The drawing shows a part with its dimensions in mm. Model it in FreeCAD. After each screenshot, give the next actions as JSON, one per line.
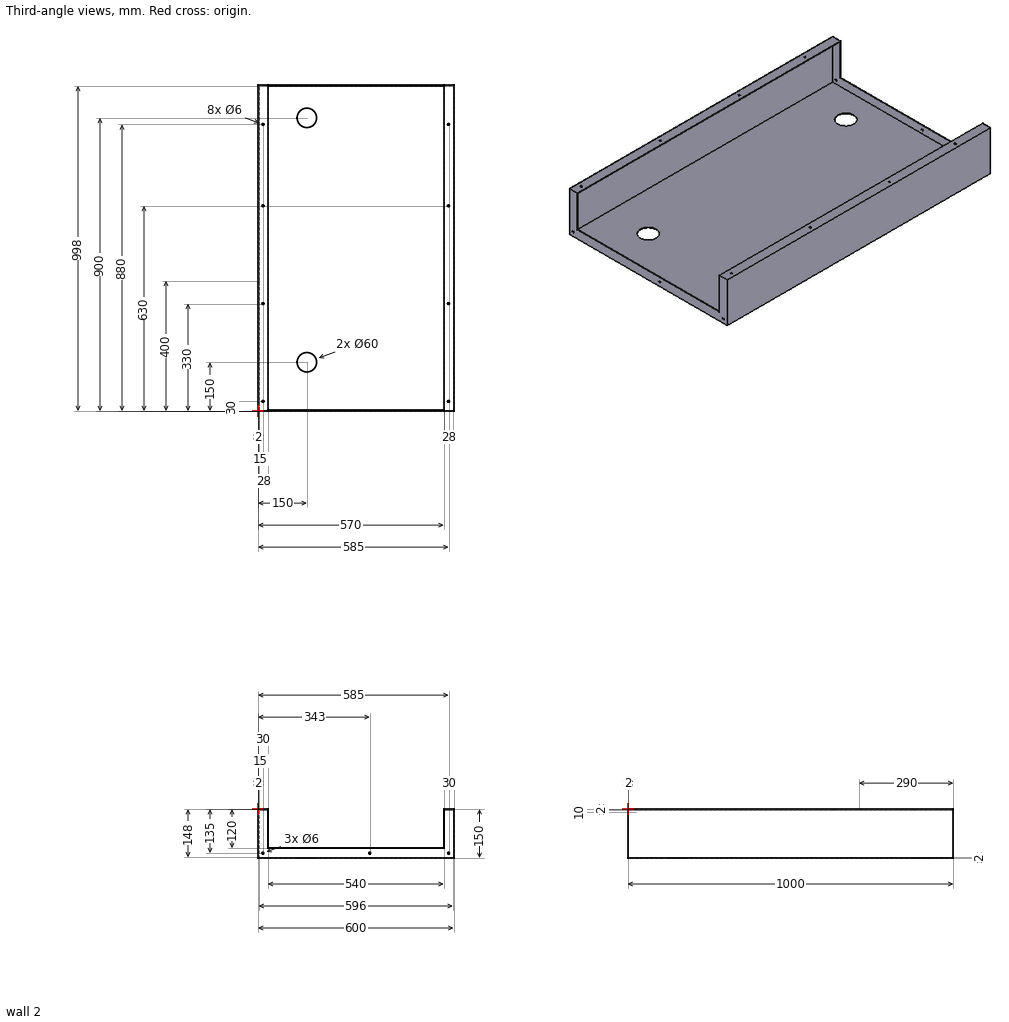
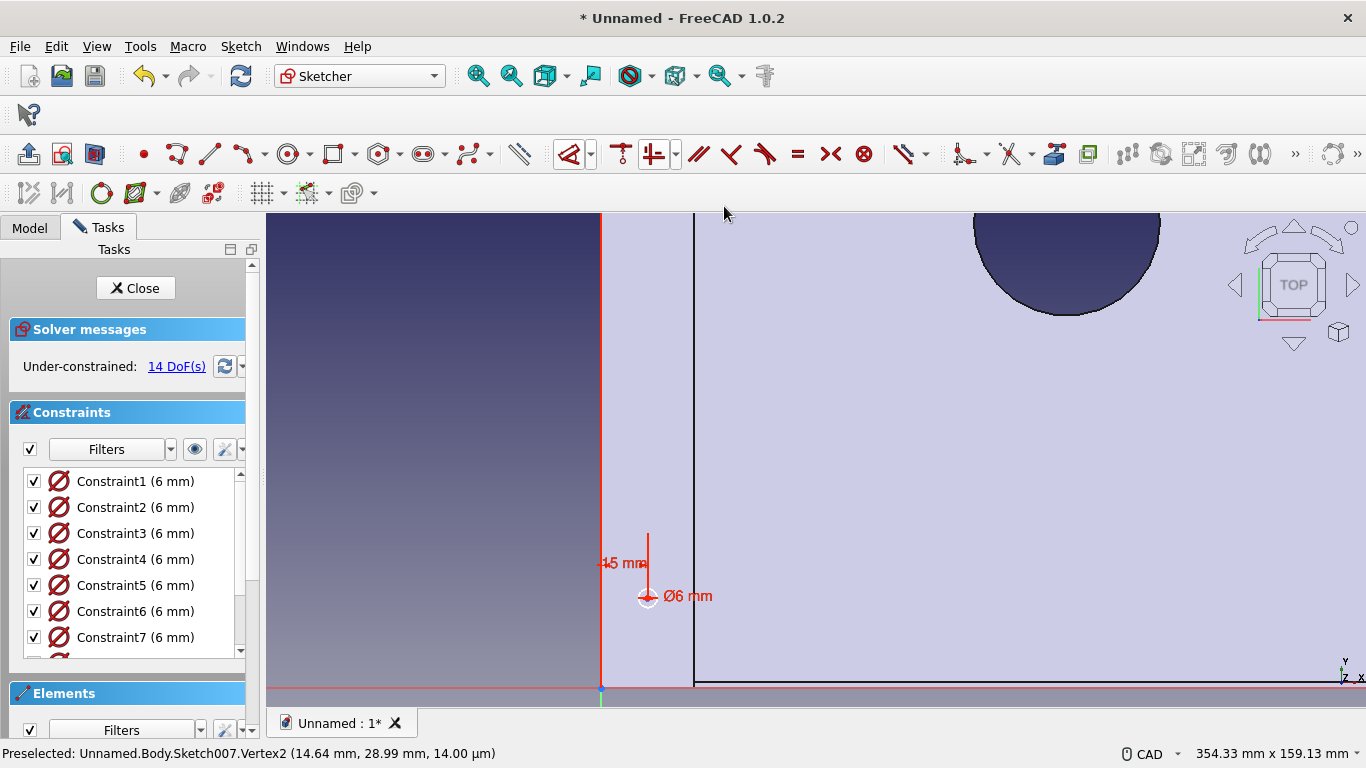
{"action": "left_click", "coordinate": [648, 598]}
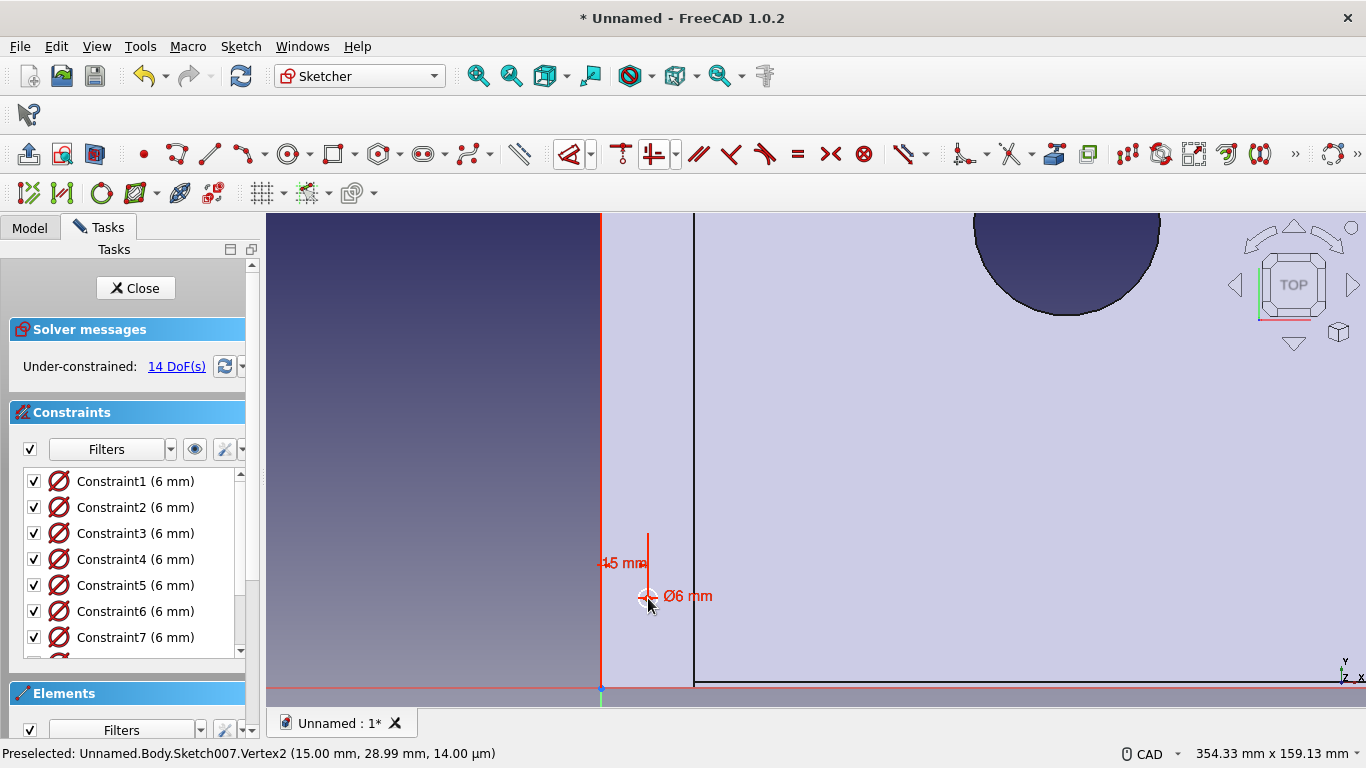
{"action": "left_click", "coordinate": [590, 154]}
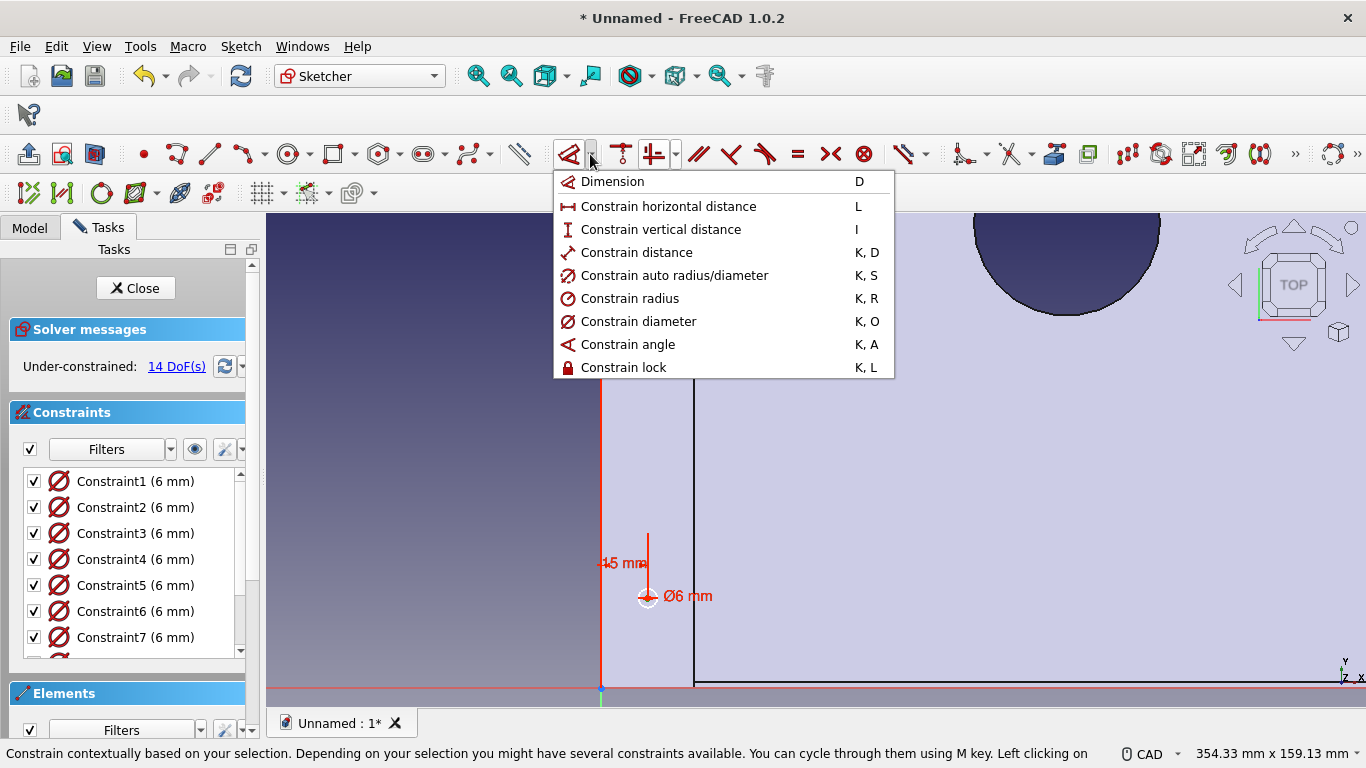
{"action": "left_click", "coordinate": [724, 230]}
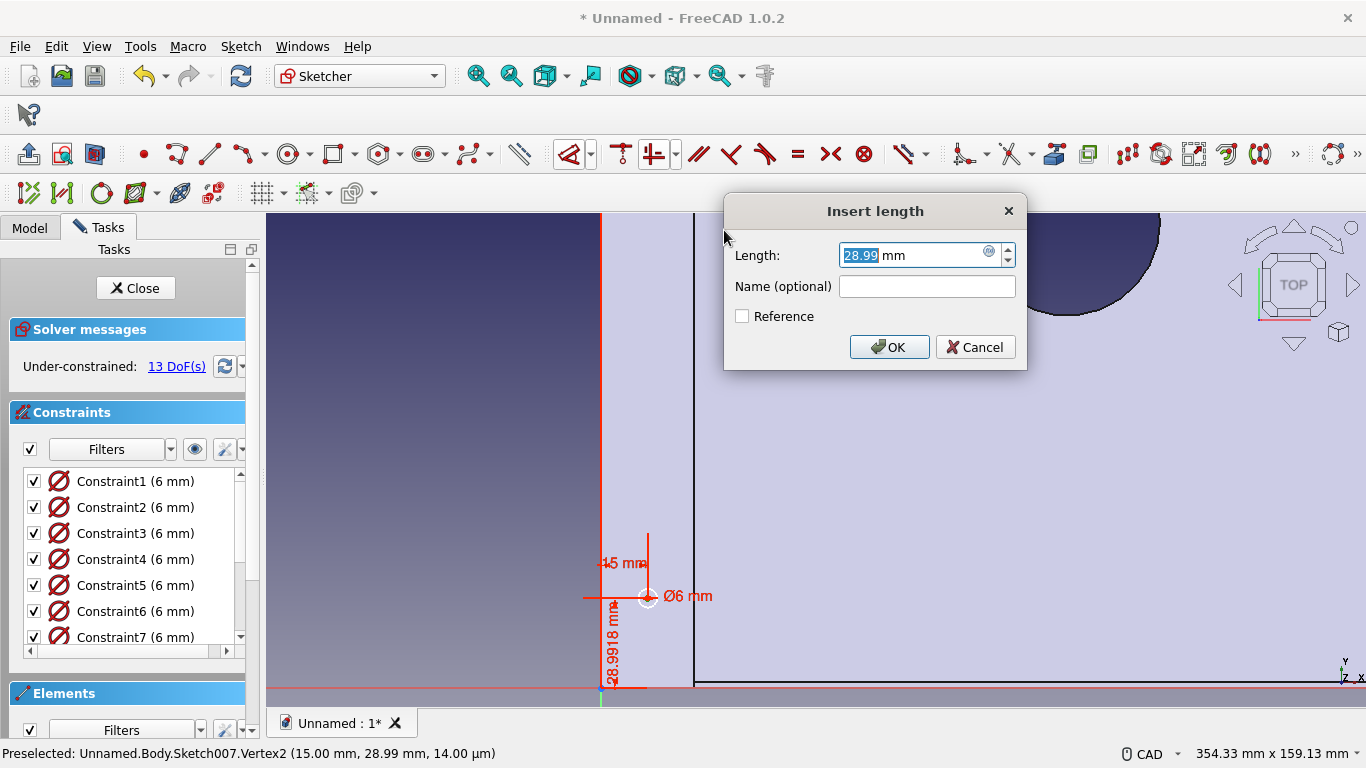
{"action": "type", "text": "30"}
{"action": "key", "text": "Return"}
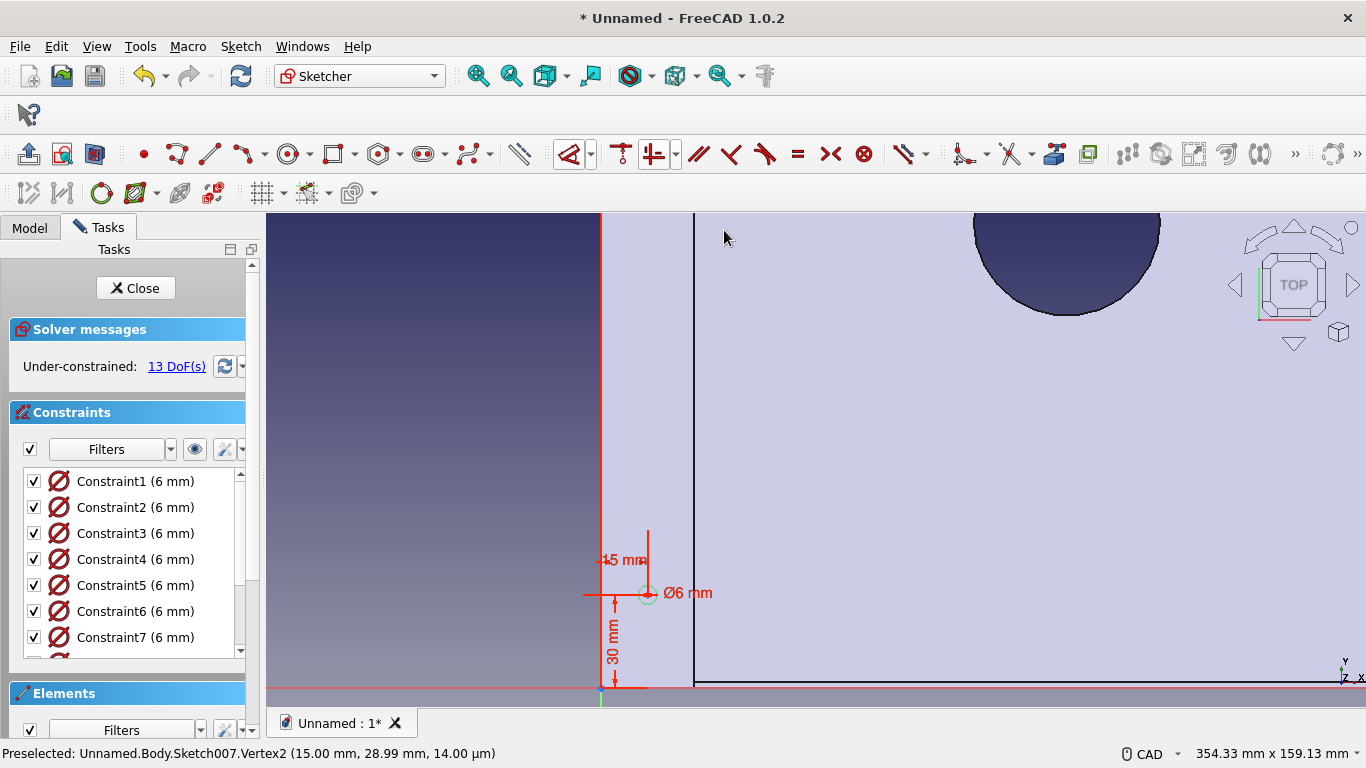
{"action": "scroll", "coordinate": [652, 602], "scroll_direction": "down", "scroll_amount": 11}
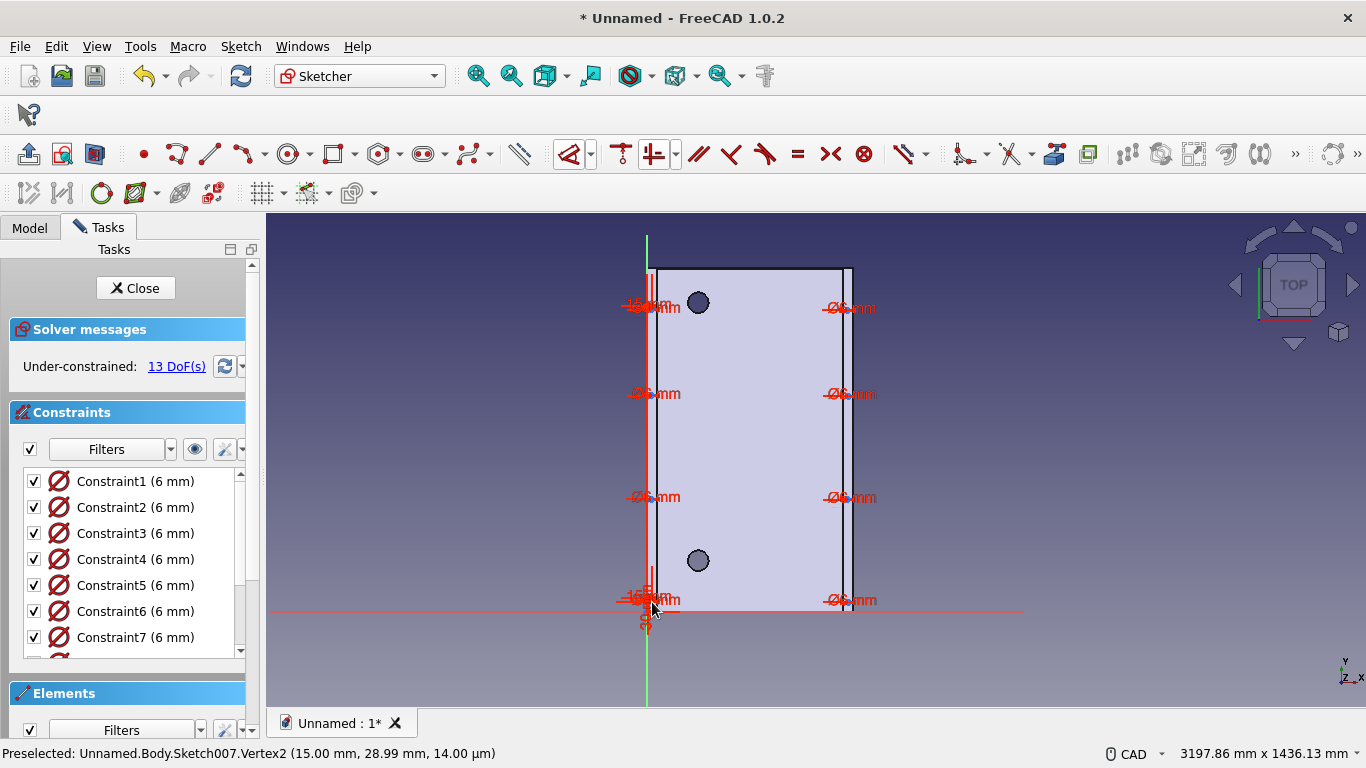
{"action": "scroll", "coordinate": [652, 499], "scroll_direction": "up", "scroll_amount": 11}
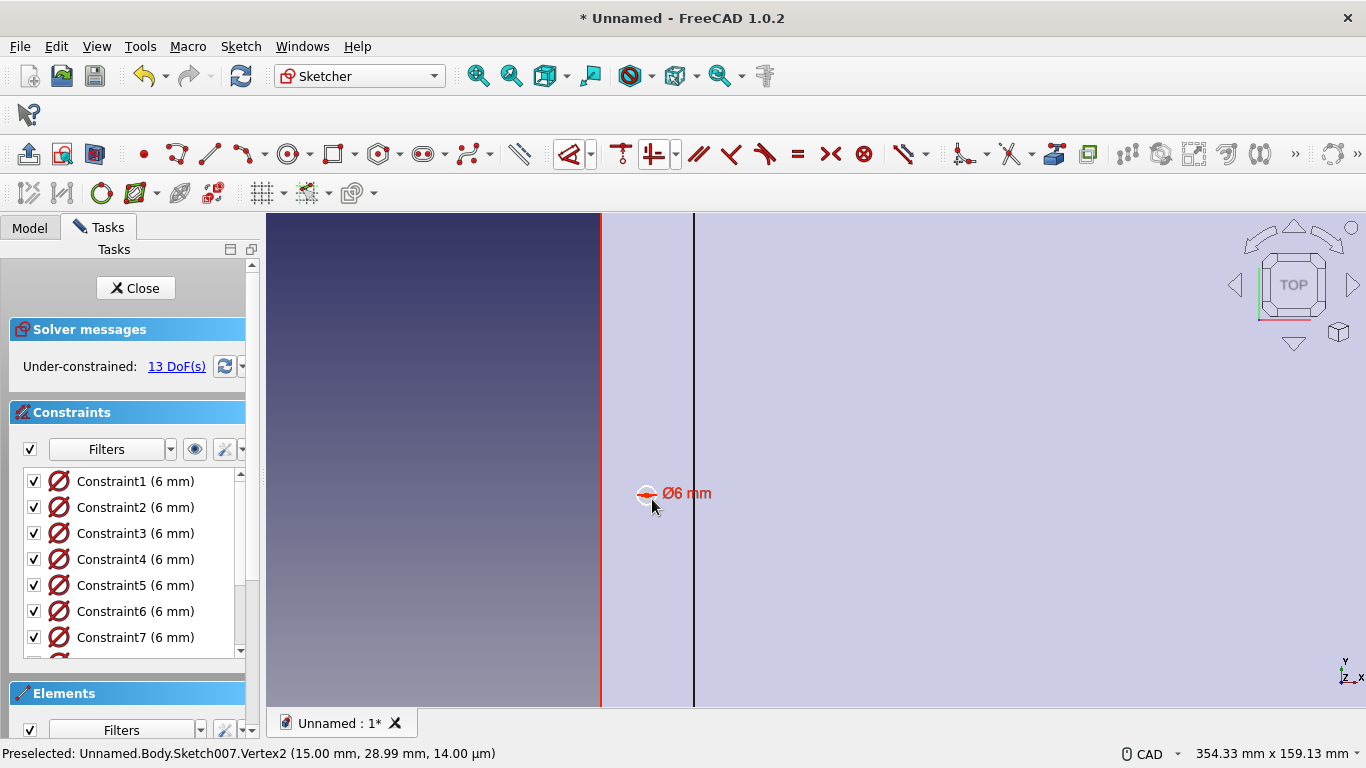
{"action": "left_click", "coordinate": [647, 495]}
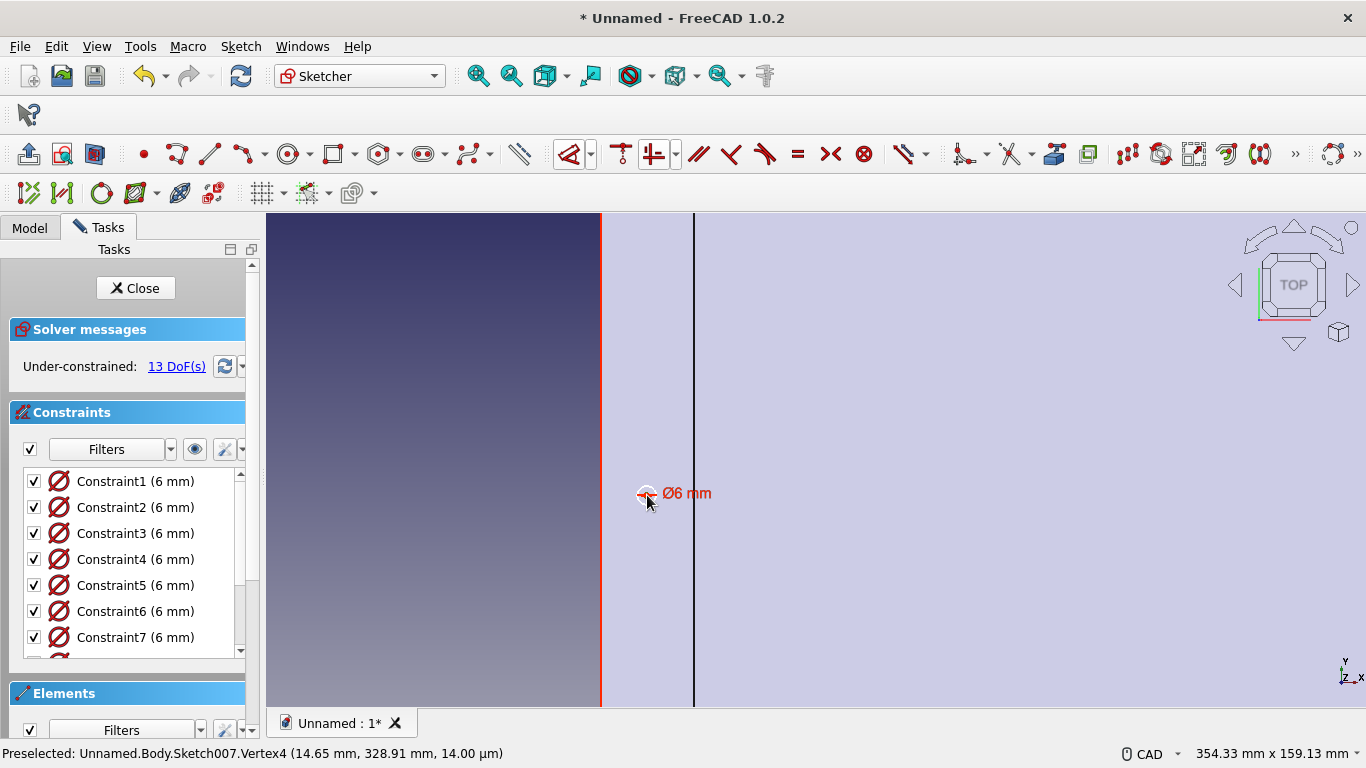
{"action": "left_click", "coordinate": [590, 154]}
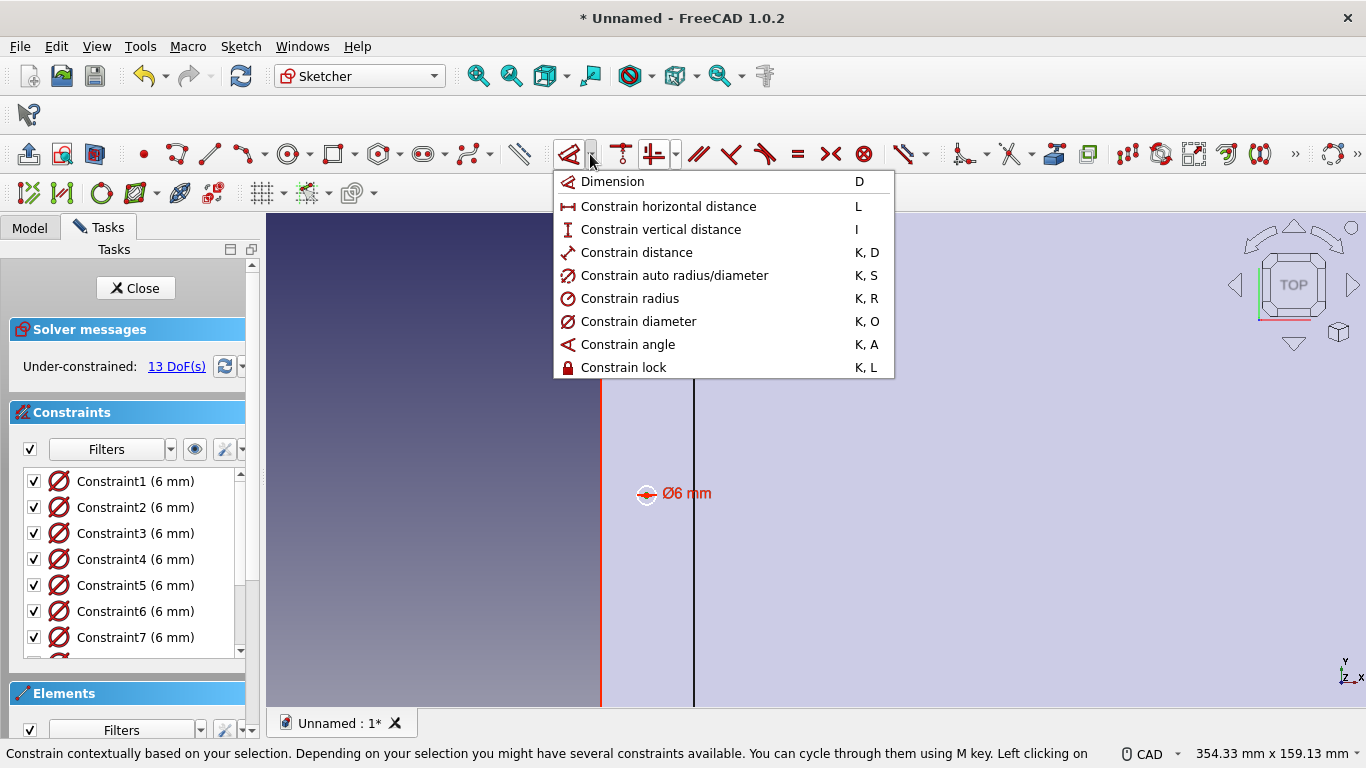
{"action": "left_click", "coordinate": [724, 206]}